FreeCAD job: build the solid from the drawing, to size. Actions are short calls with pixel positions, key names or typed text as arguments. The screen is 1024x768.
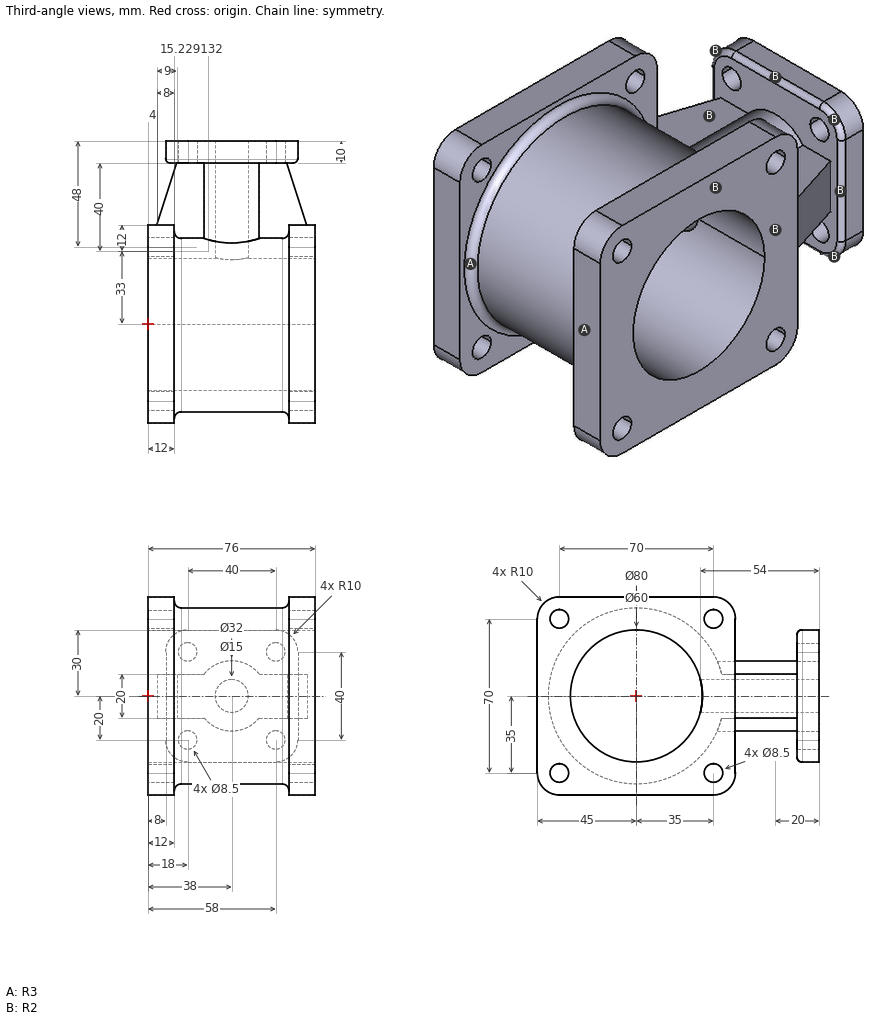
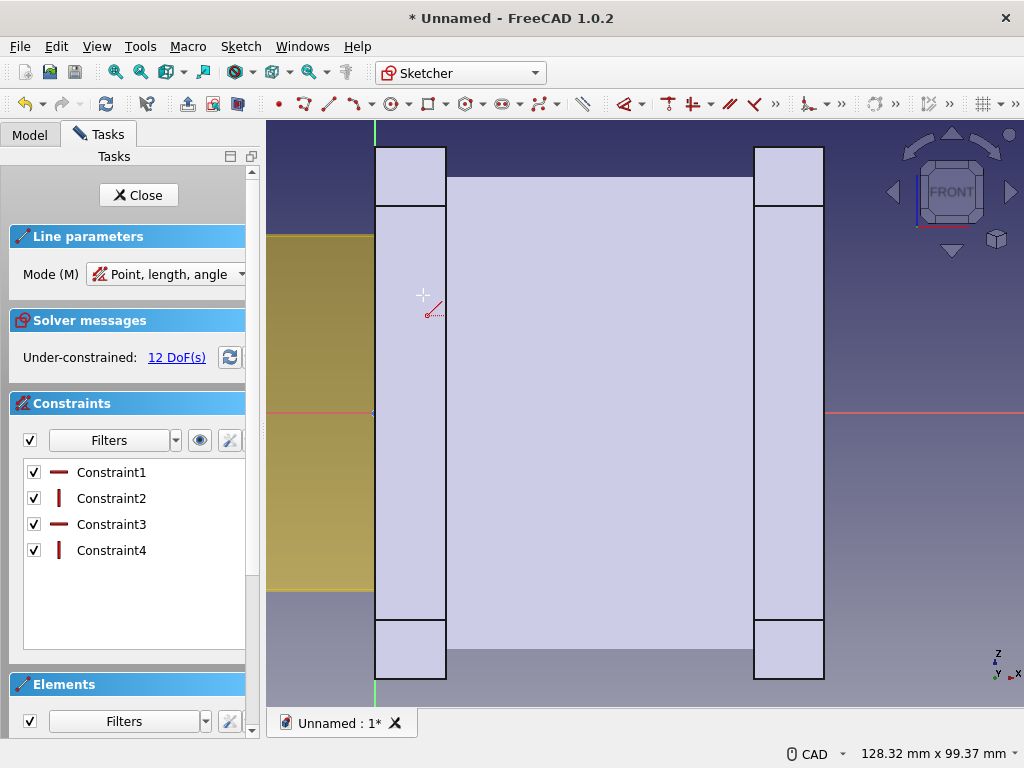
key(g)
key(3)
key(a)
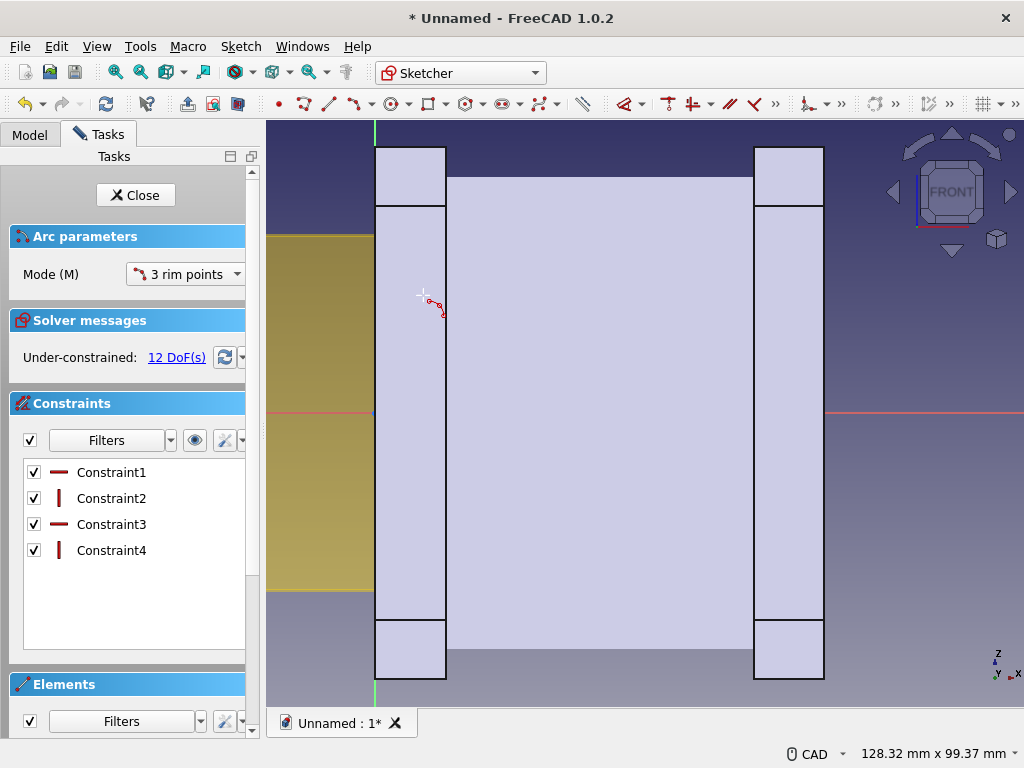
click(718, 237)
click(777, 296)
click(760, 253)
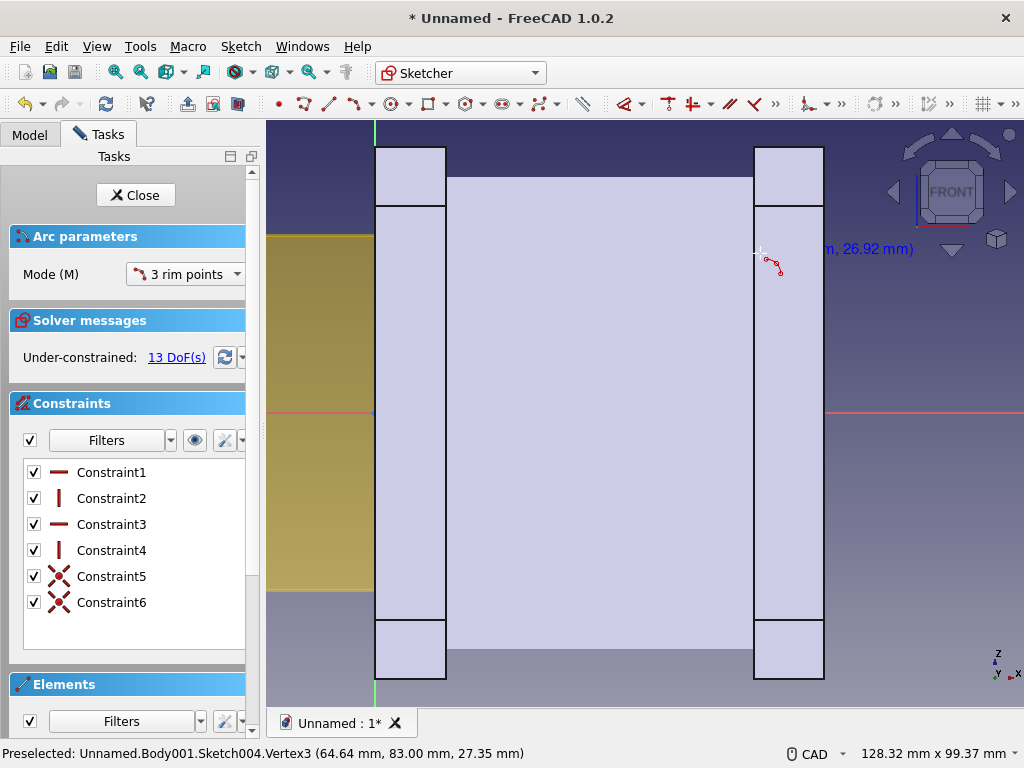
click(777, 532)
click(718, 591)
click(760, 573)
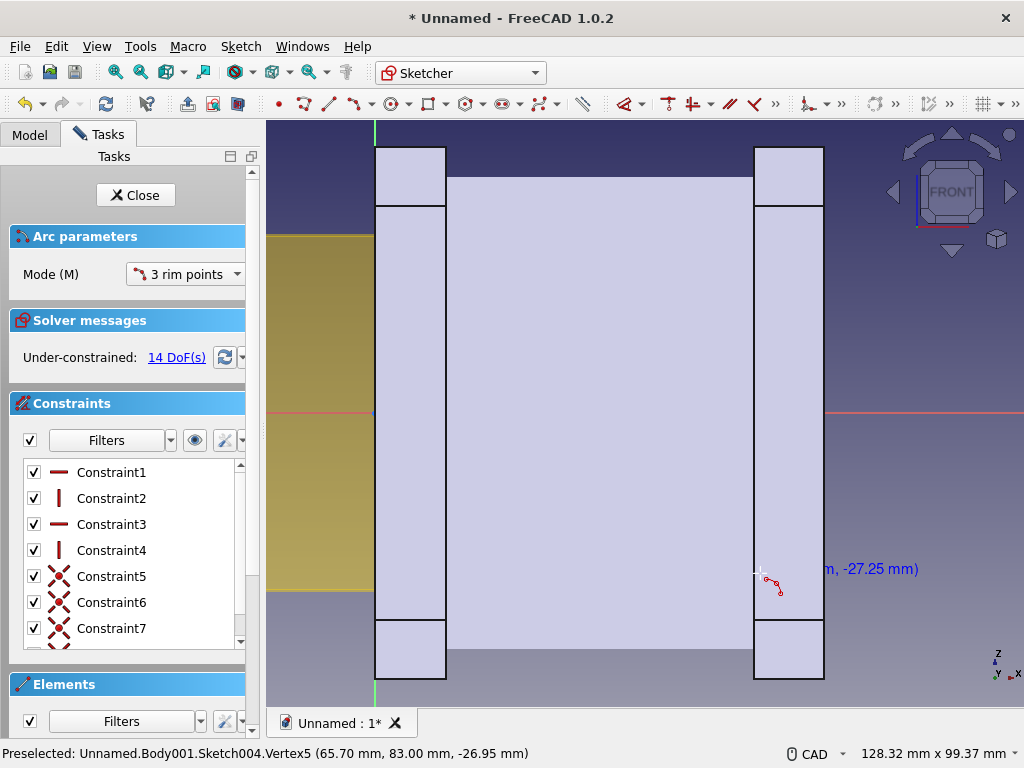
click(482, 591)
click(423, 532)
click(440, 573)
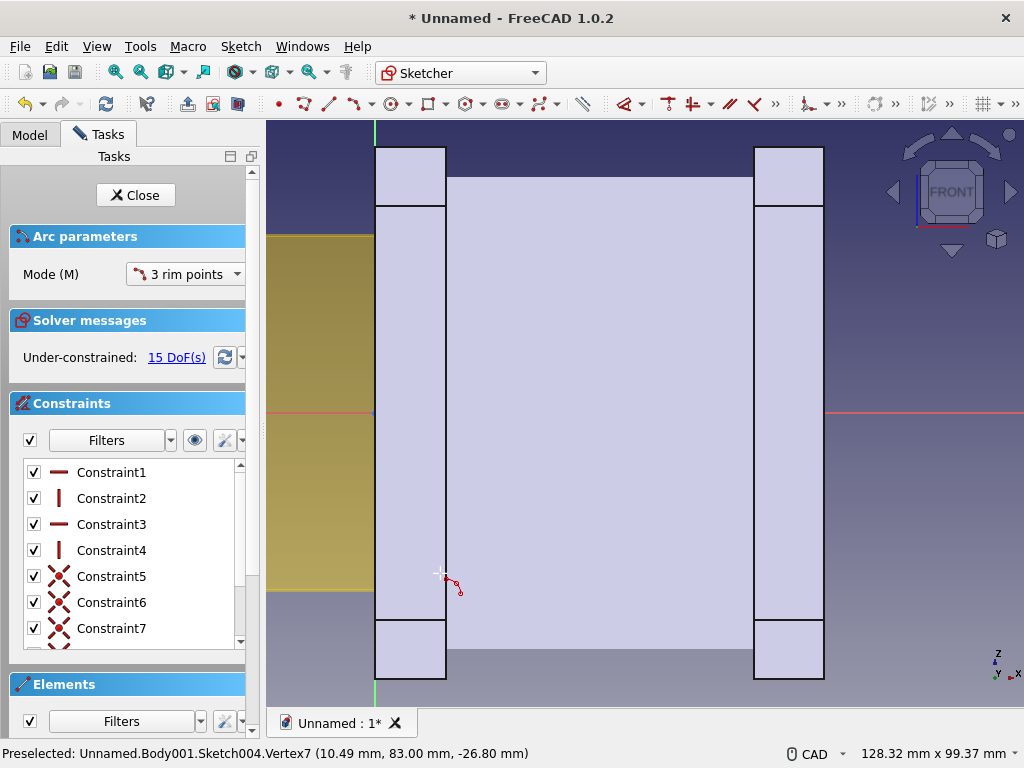
click(423, 296)
click(482, 237)
click(440, 253)
key(Escape)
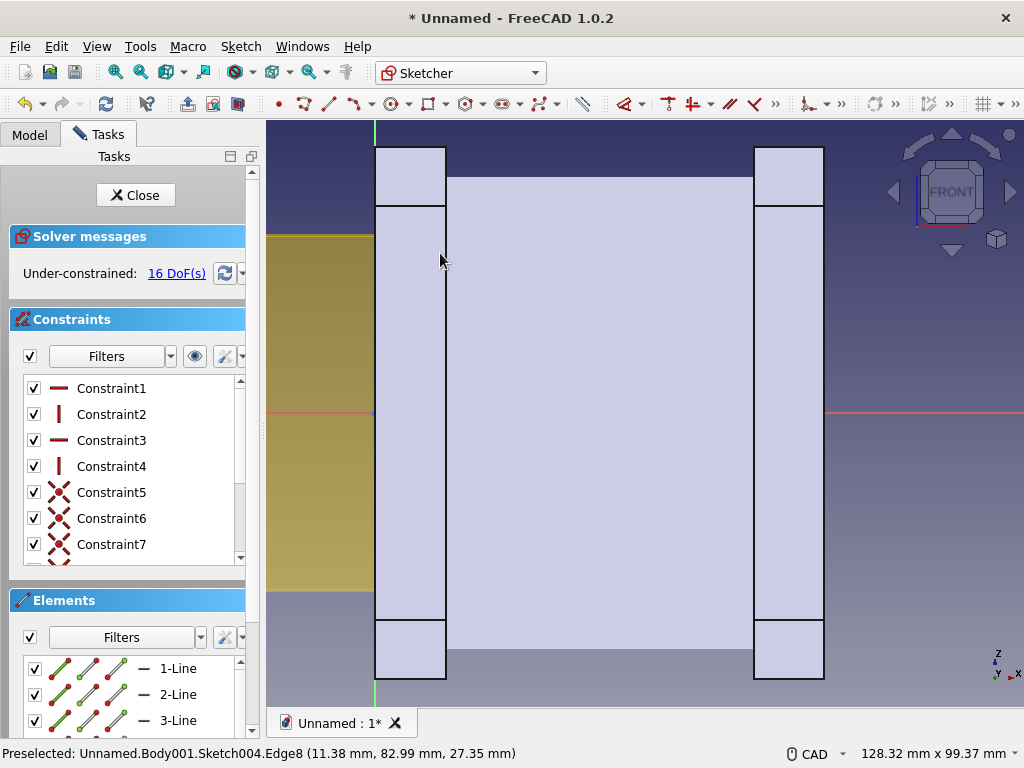
click(553, 237)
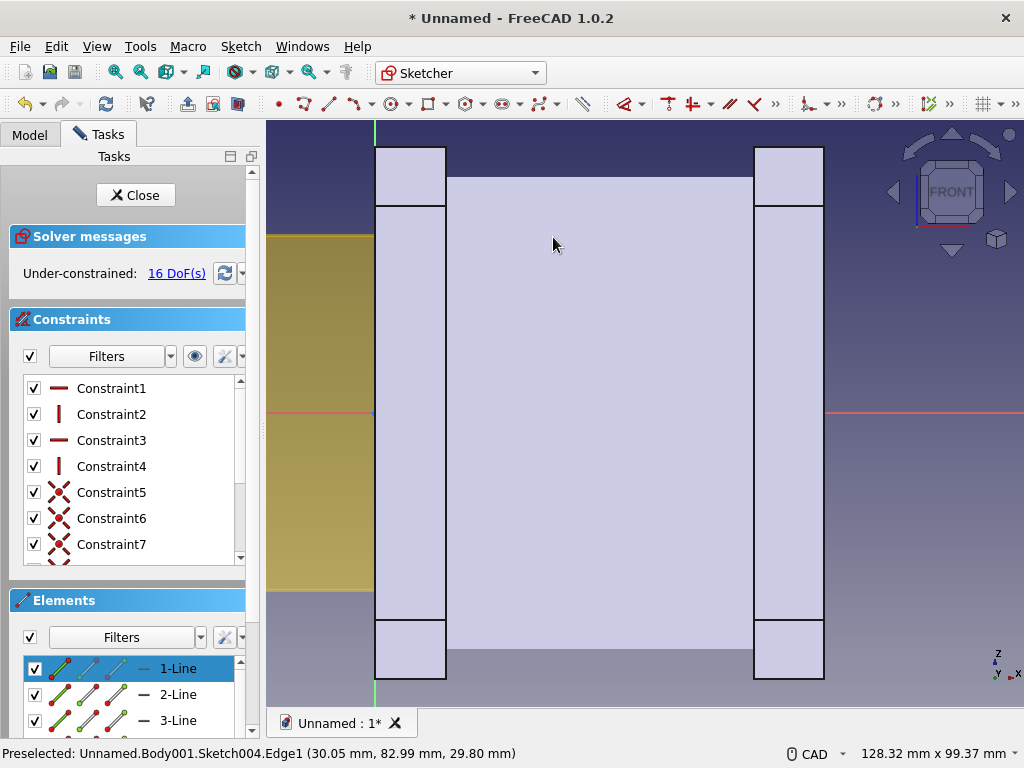
click(771, 269)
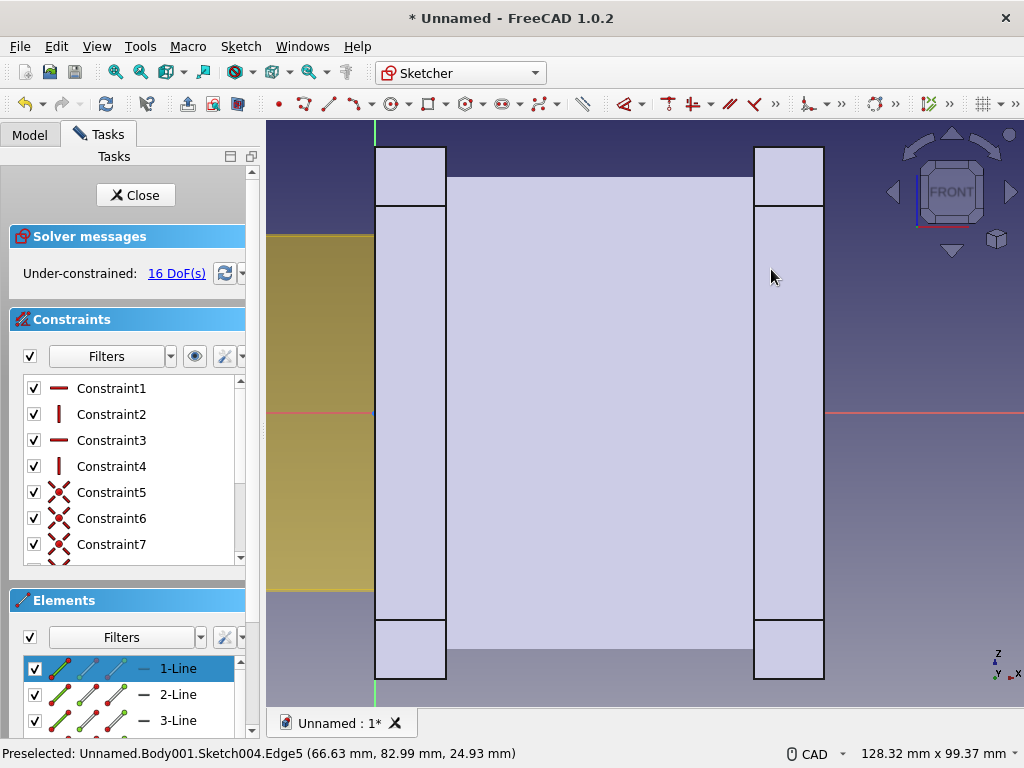
key(t)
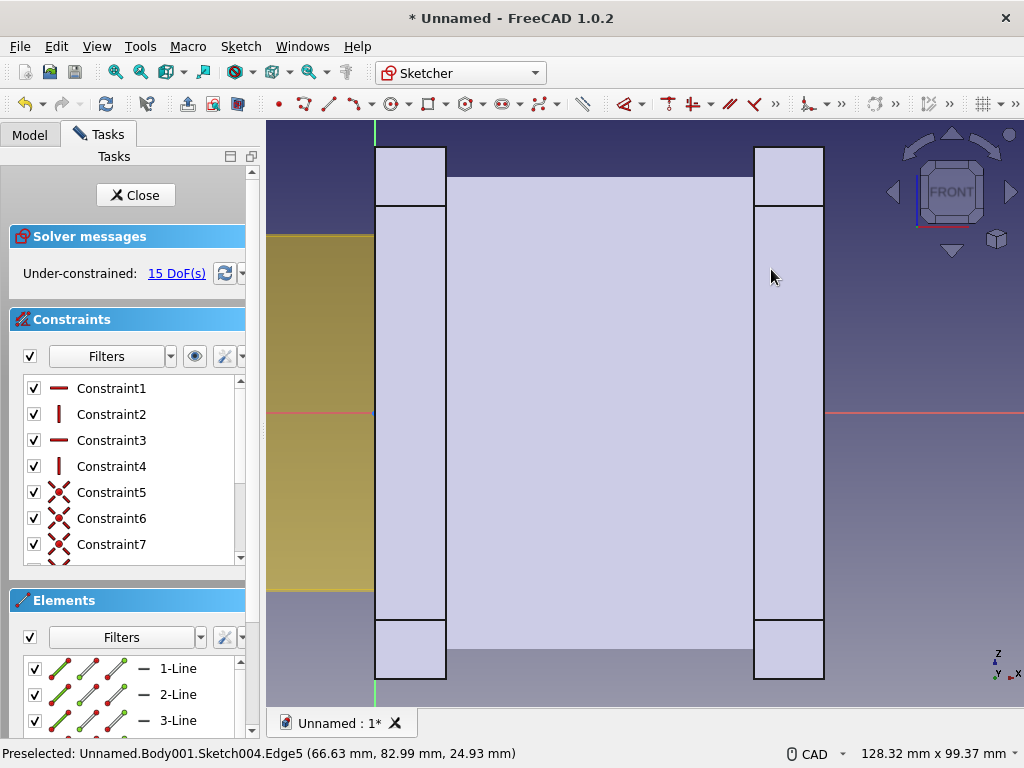
click(553, 237)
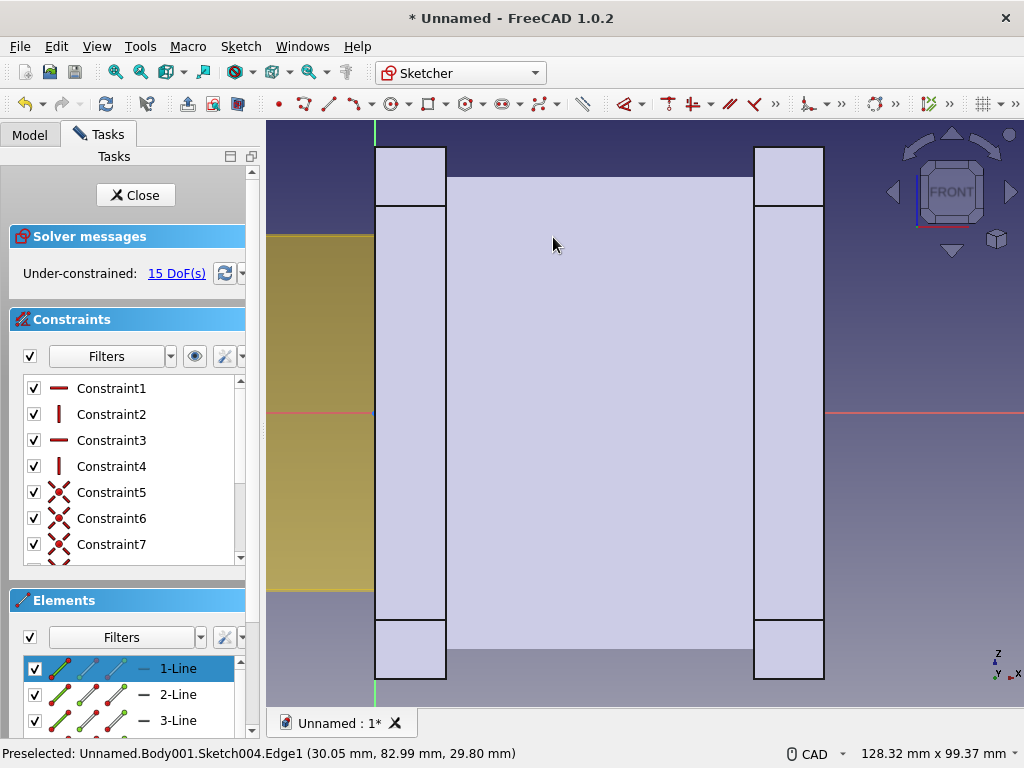
click(455, 243)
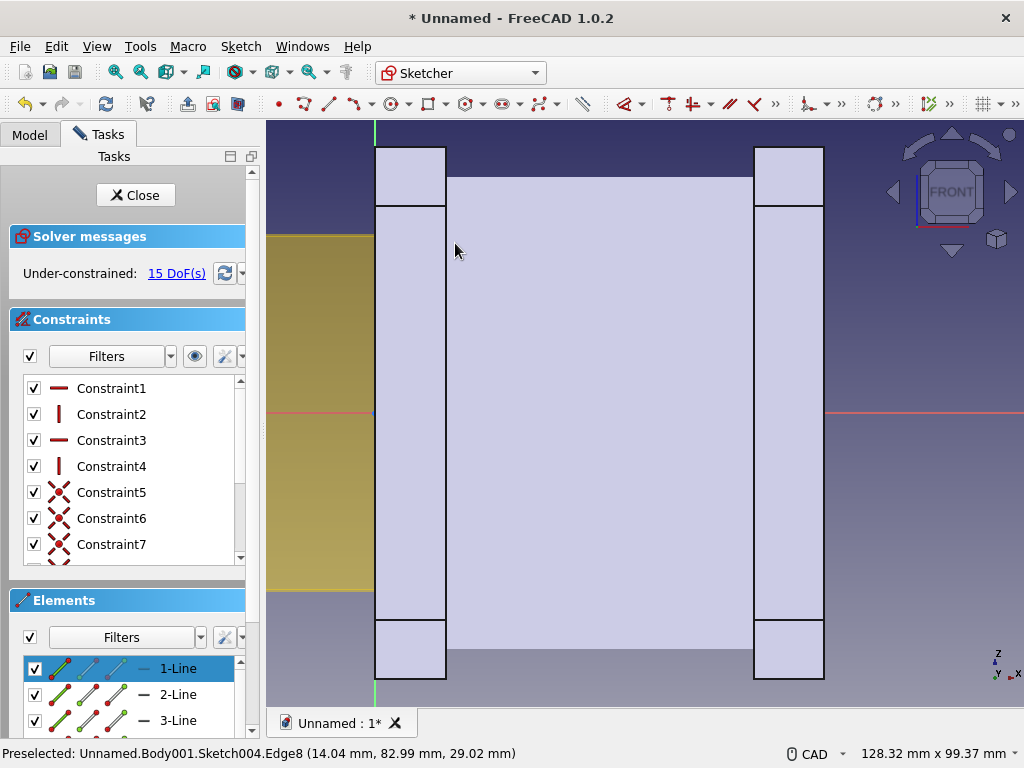
key(t)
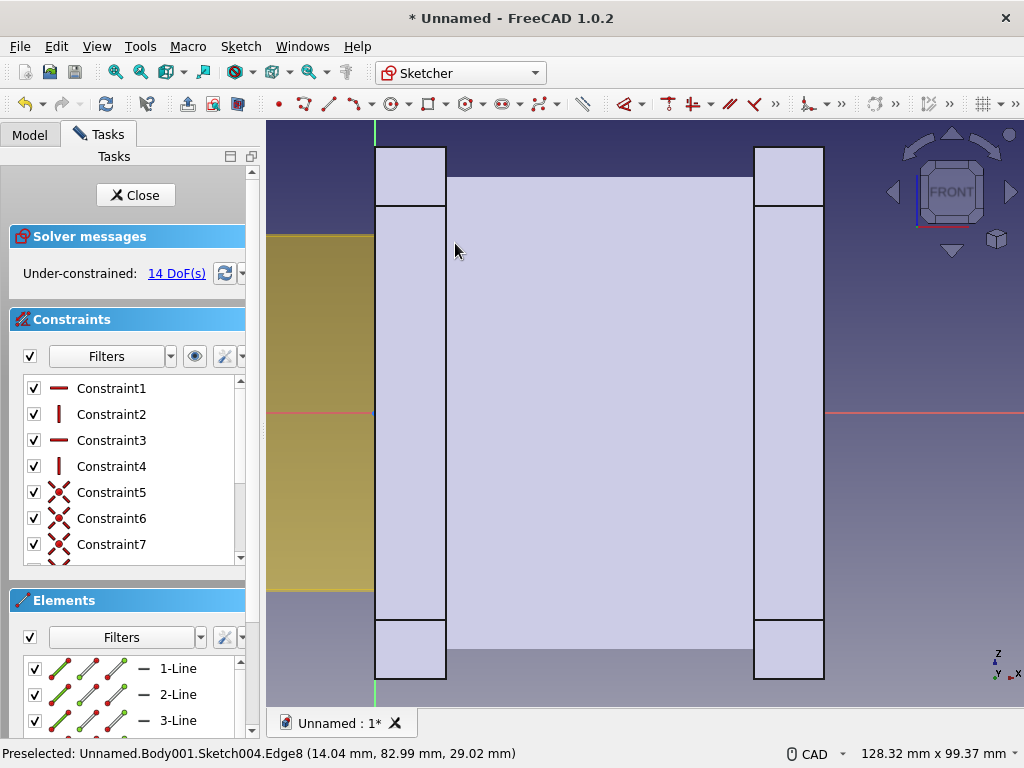
click(777, 367)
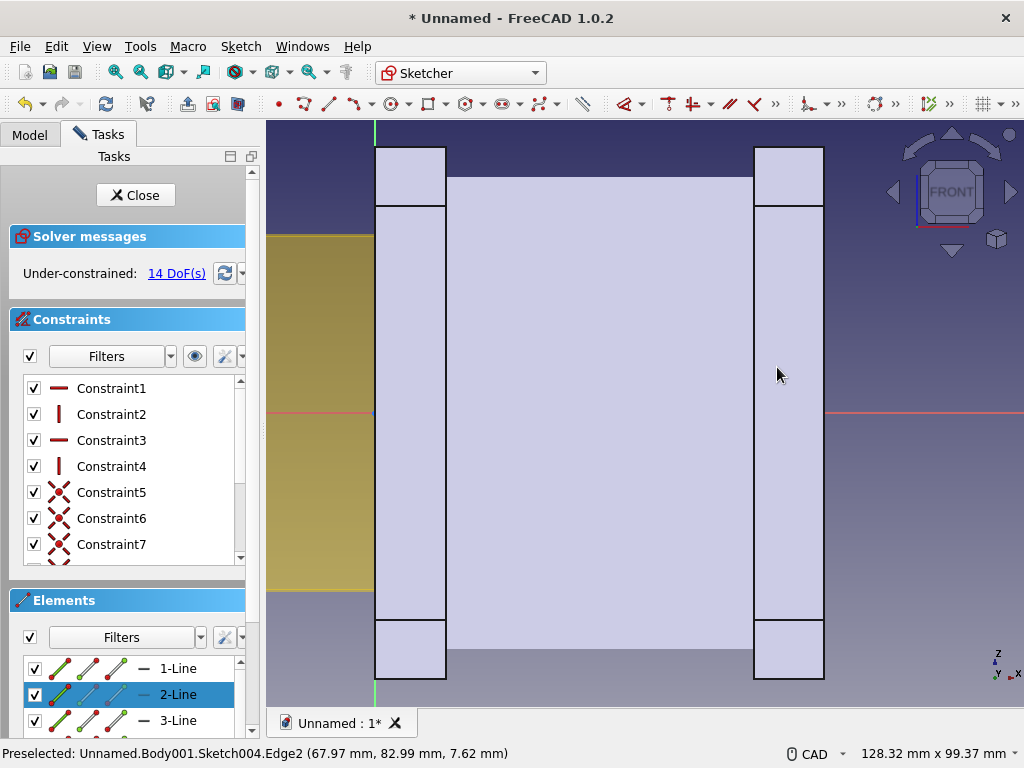
click(771, 269)